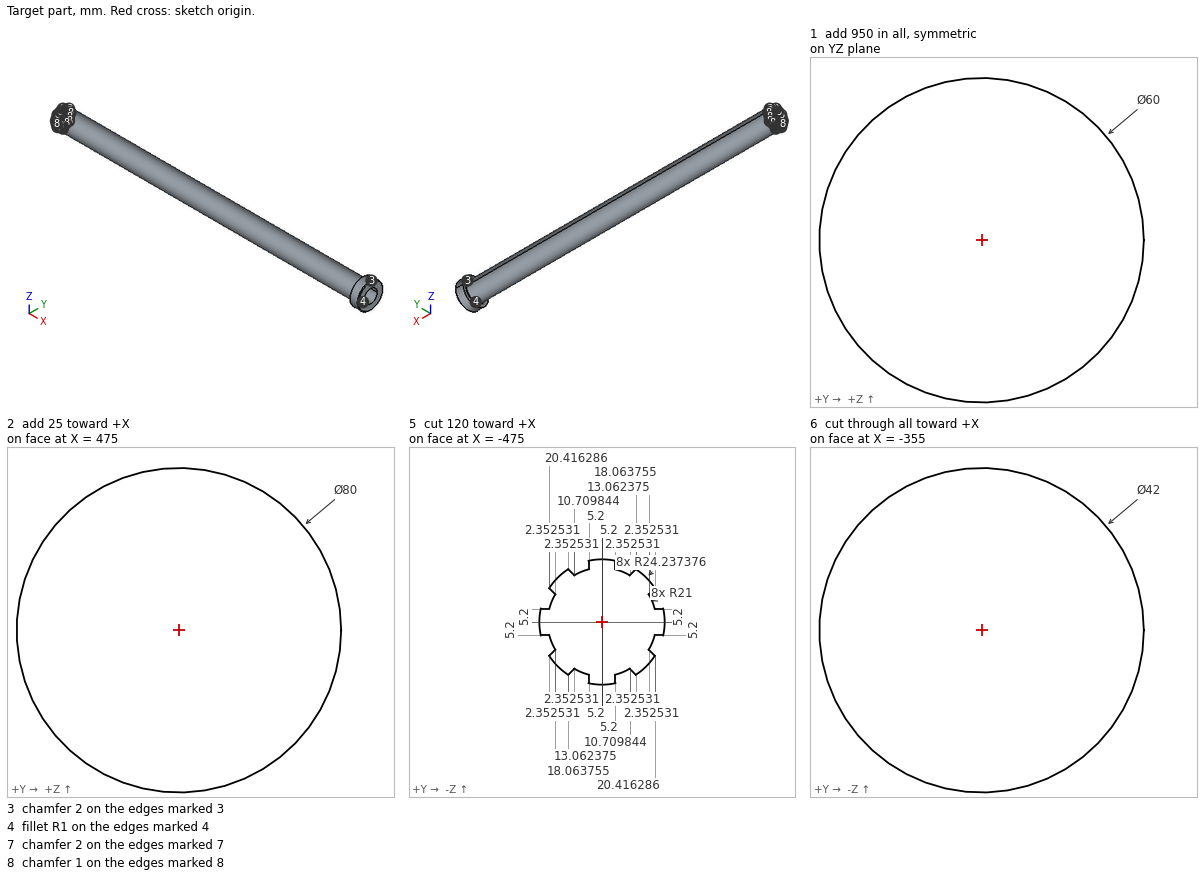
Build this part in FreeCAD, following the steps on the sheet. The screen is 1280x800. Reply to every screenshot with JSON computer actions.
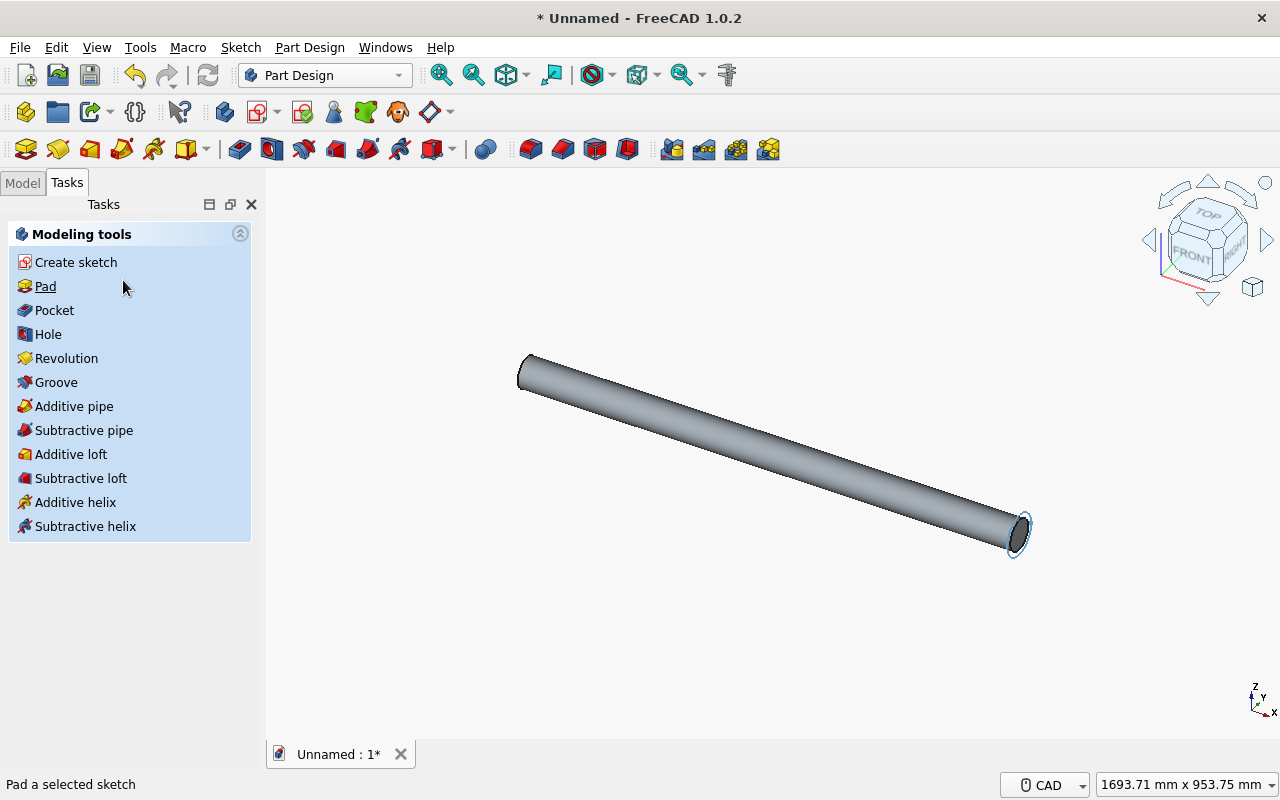
{"action": "left_click", "coordinate": [26, 150]}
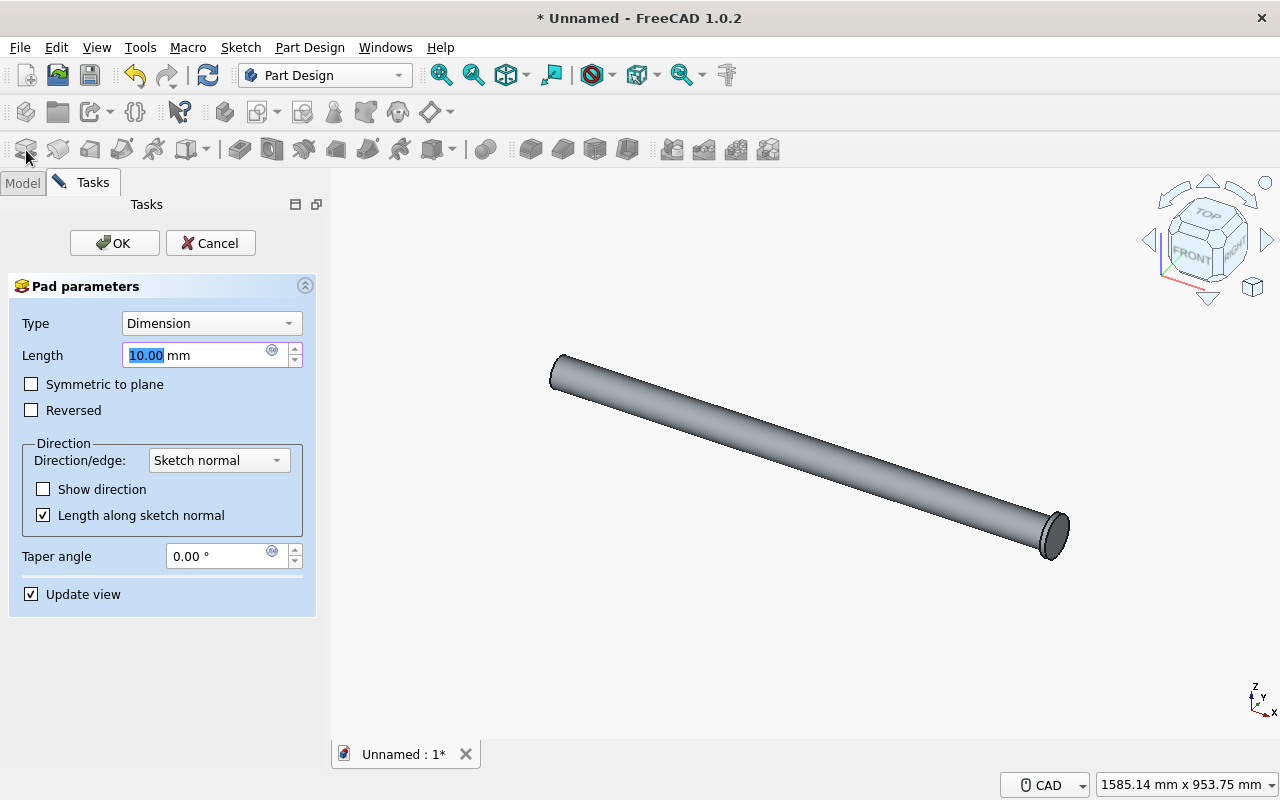
{"action": "type", "text": "25"}
{"action": "key", "text": "Tab"}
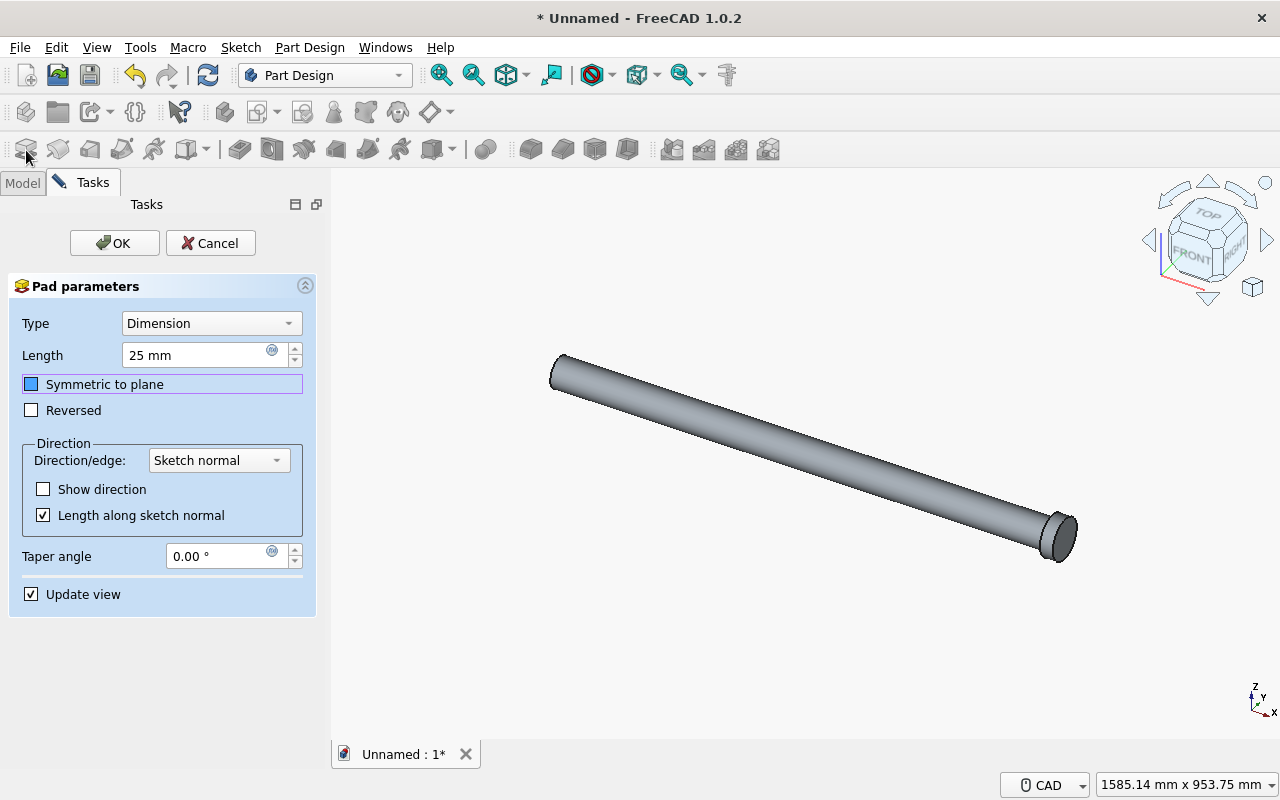
{"action": "left_click", "coordinate": [115, 243]}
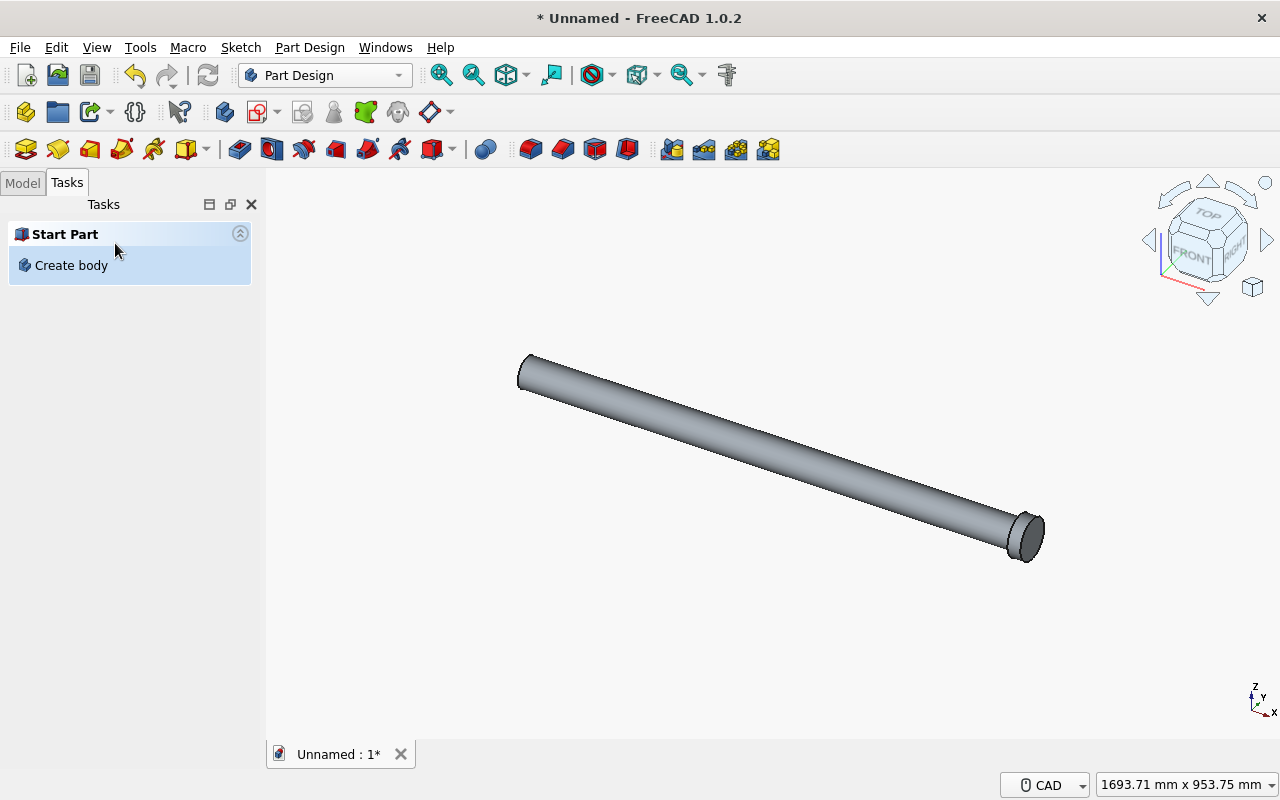
{"action": "left_click", "coordinate": [1020, 550]}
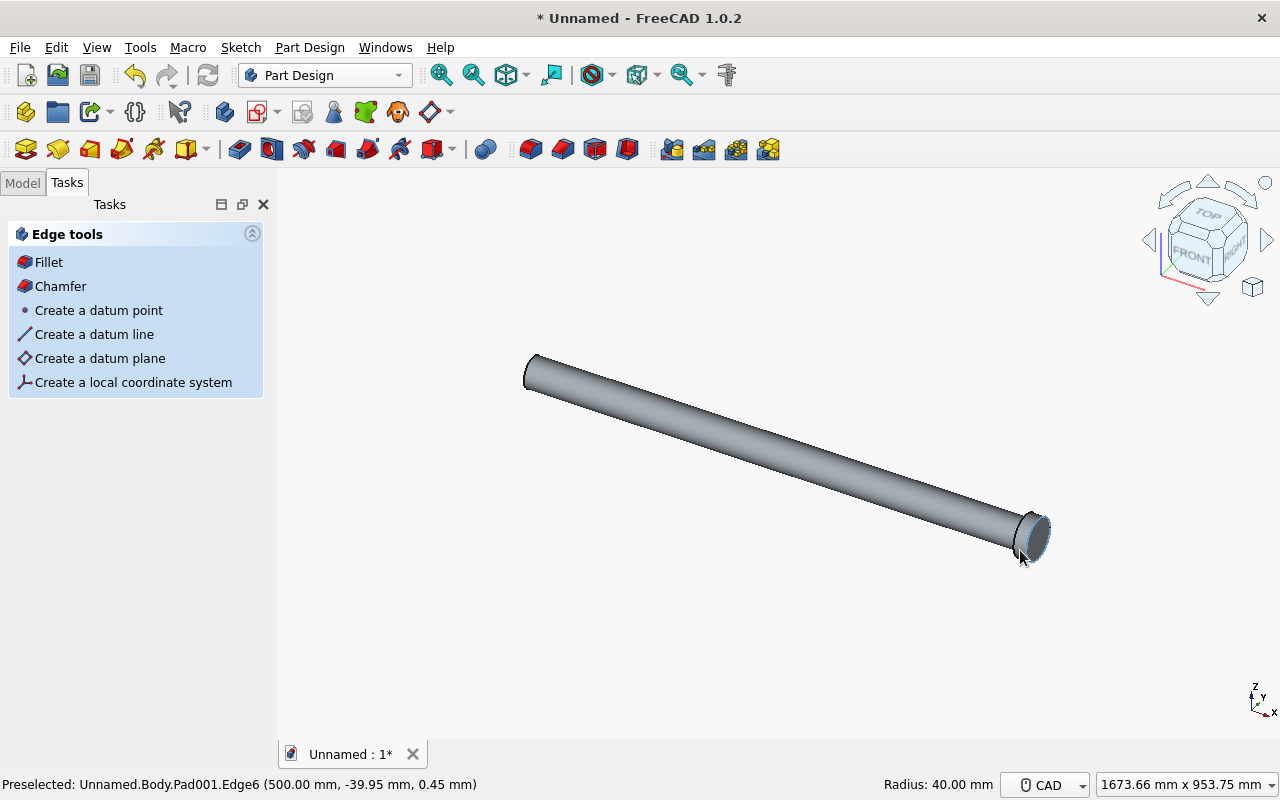
{"action": "left_click", "coordinate": [564, 150]}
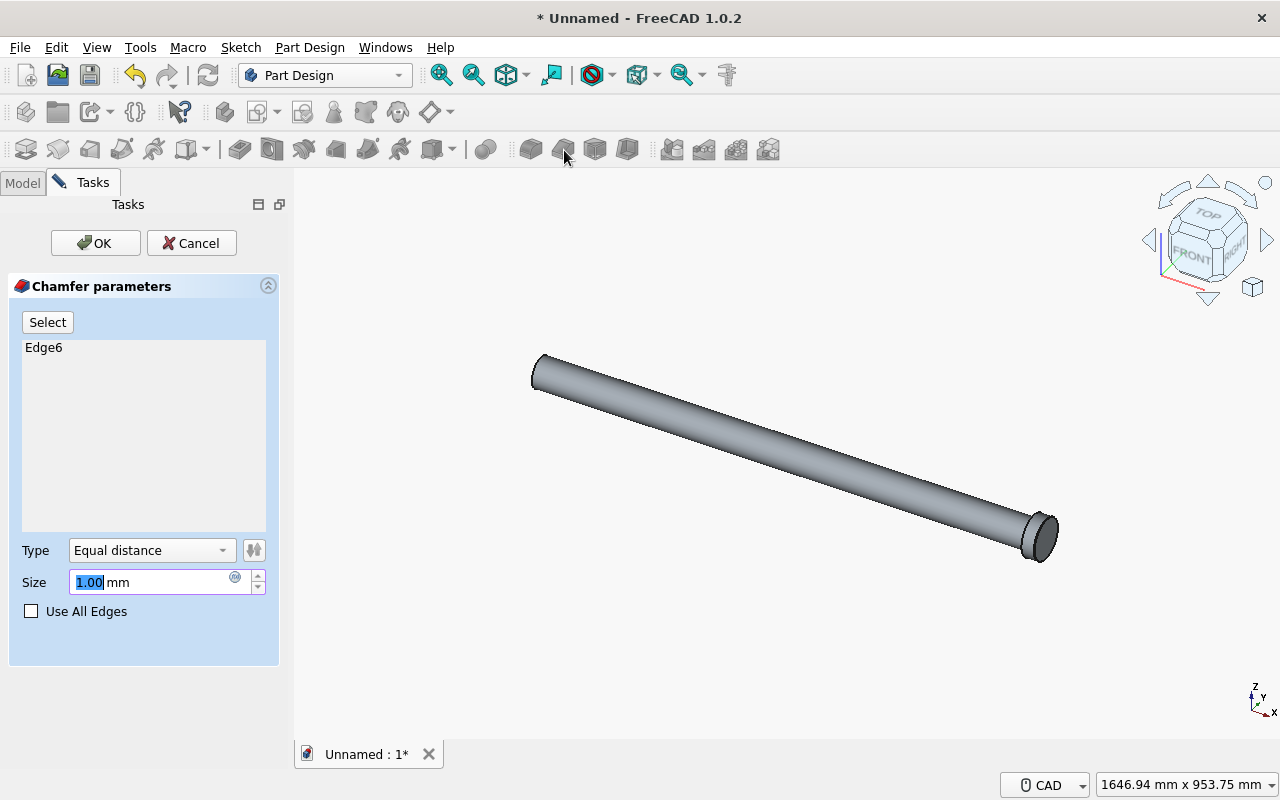
{"action": "type", "text": "2"}
{"action": "key", "text": "Tab"}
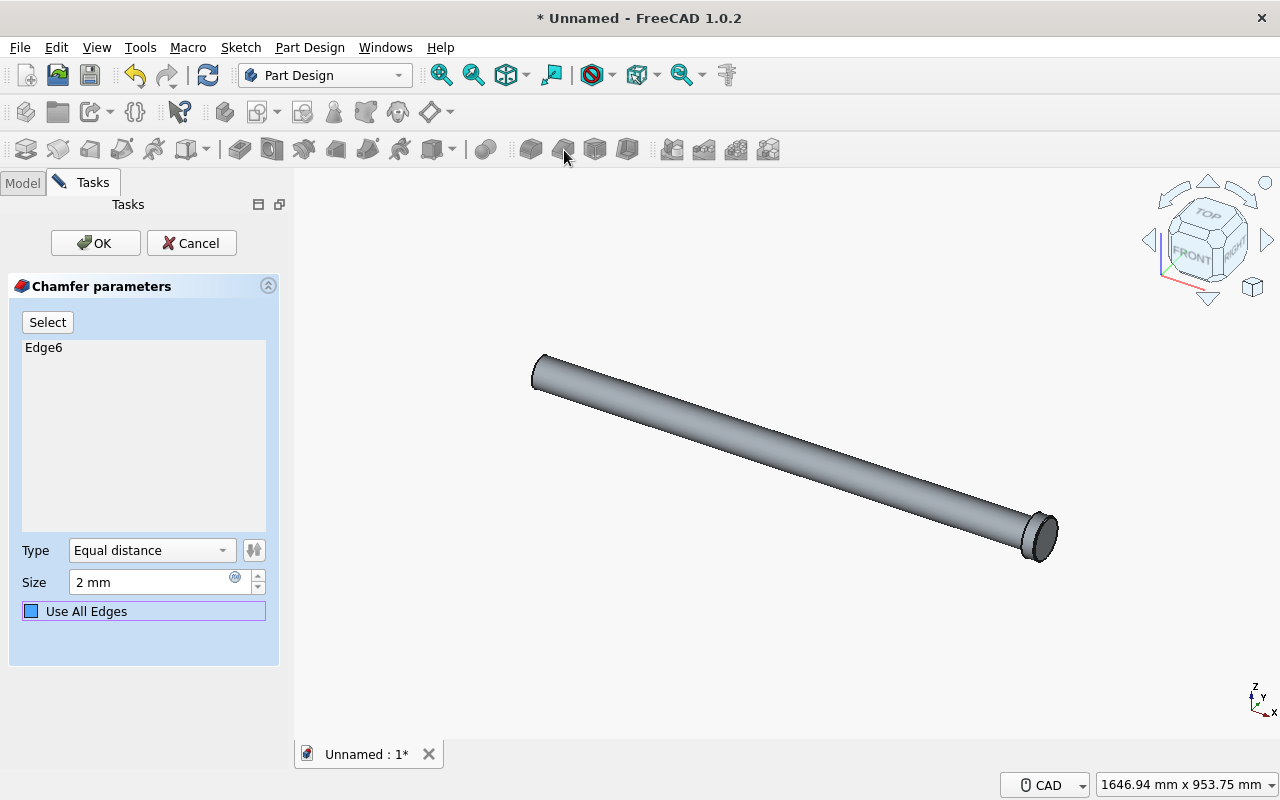
{"action": "left_click", "coordinate": [96, 243]}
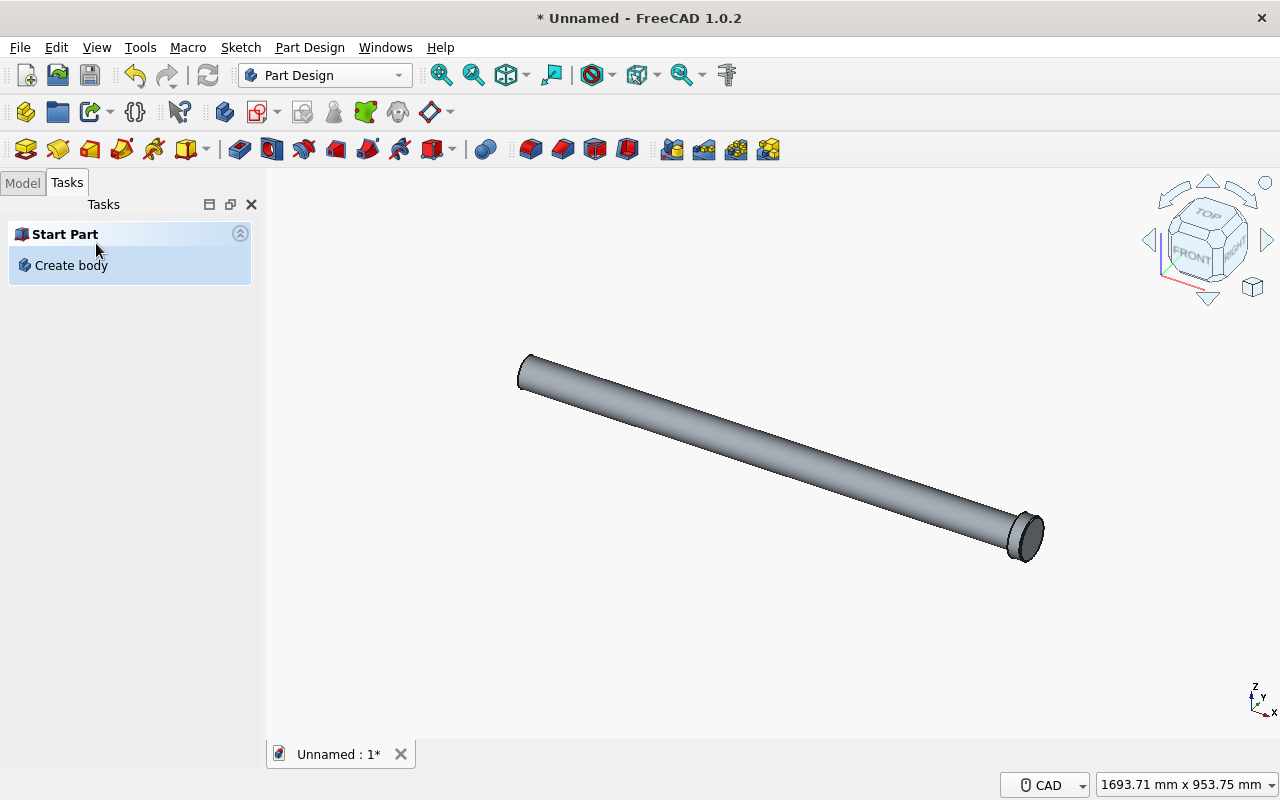
{"action": "key", "text": "0"}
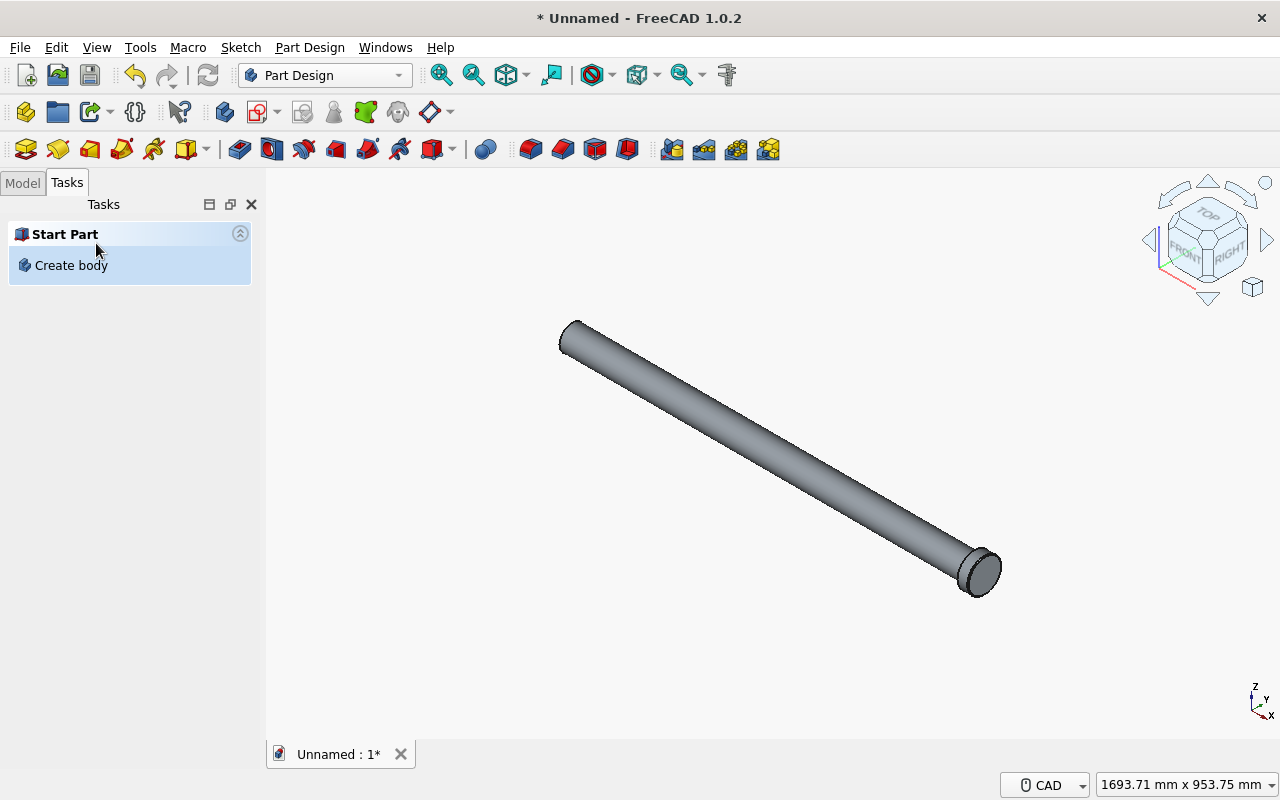
{"action": "key", "text": "2"}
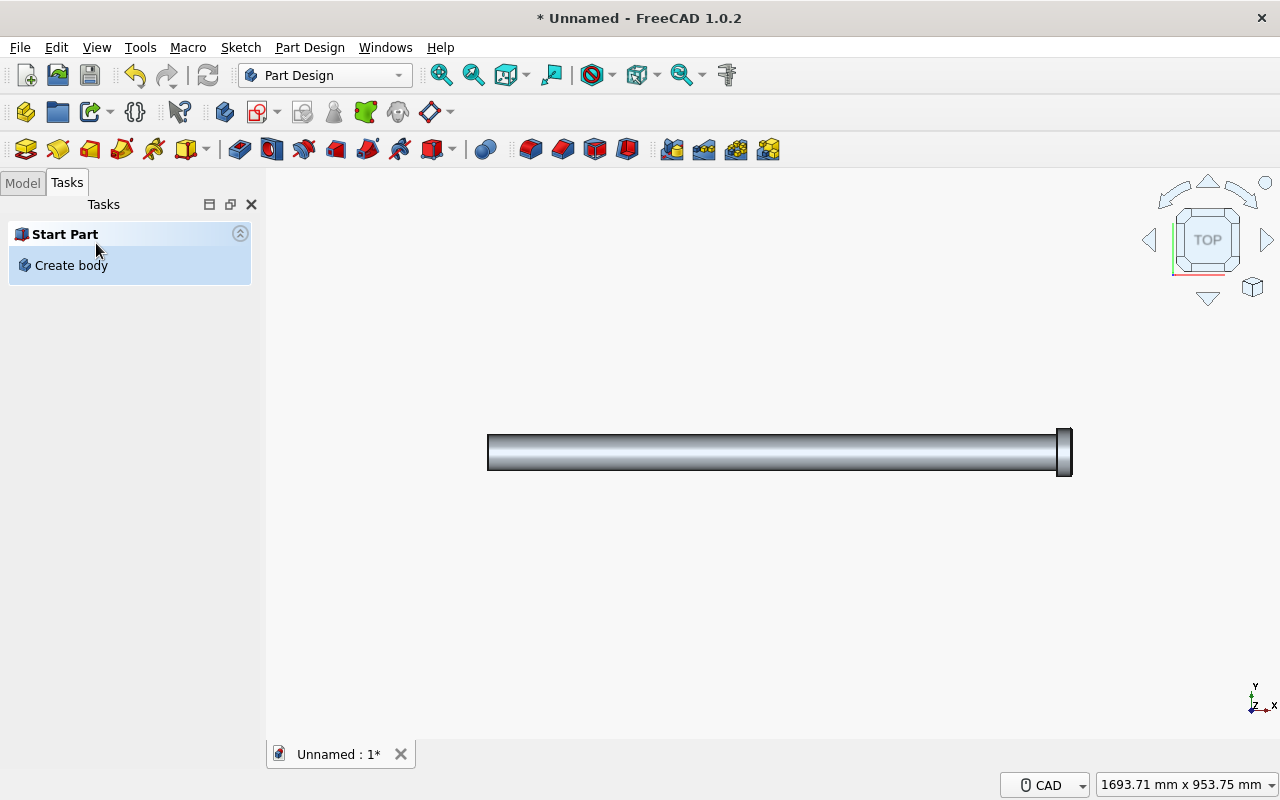
{"action": "key", "text": "1"}